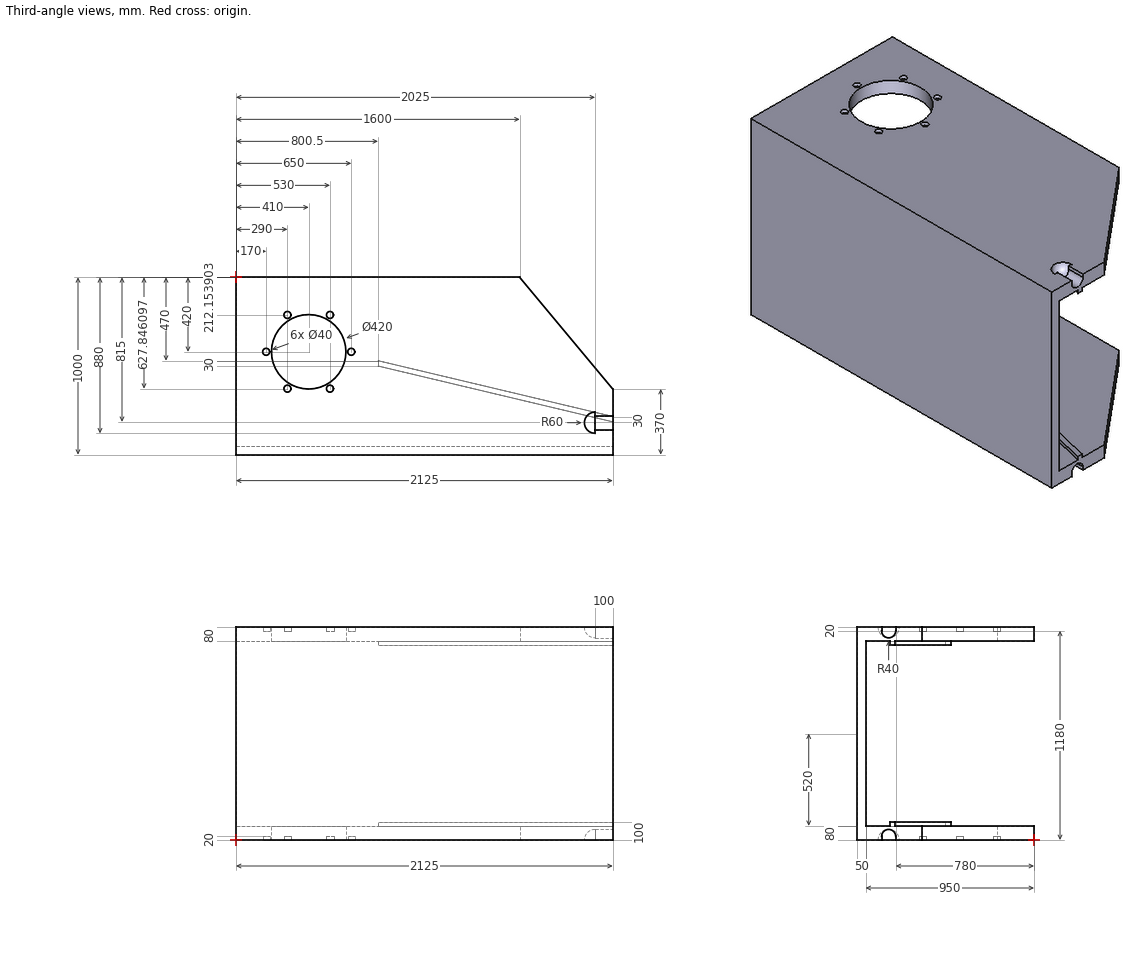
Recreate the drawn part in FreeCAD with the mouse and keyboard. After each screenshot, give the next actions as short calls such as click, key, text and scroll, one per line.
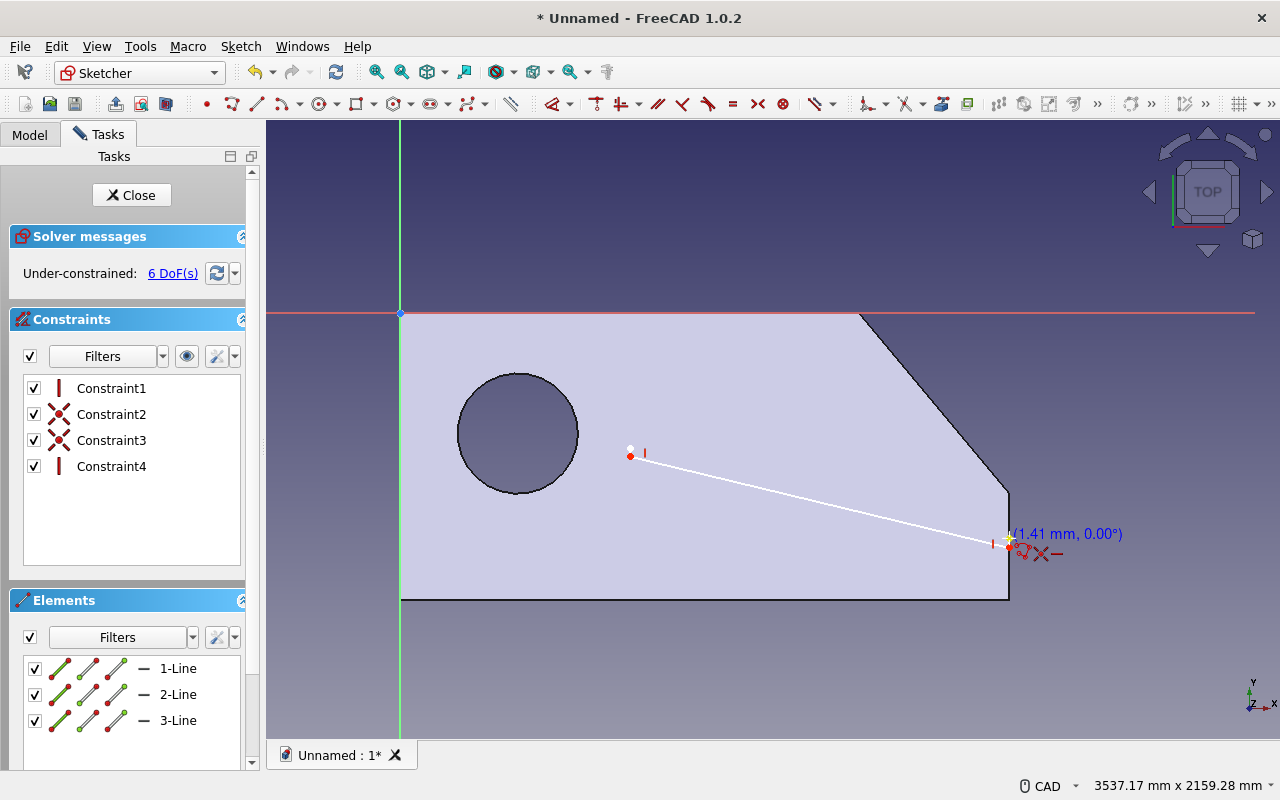
scroll(630, 448, up, 7)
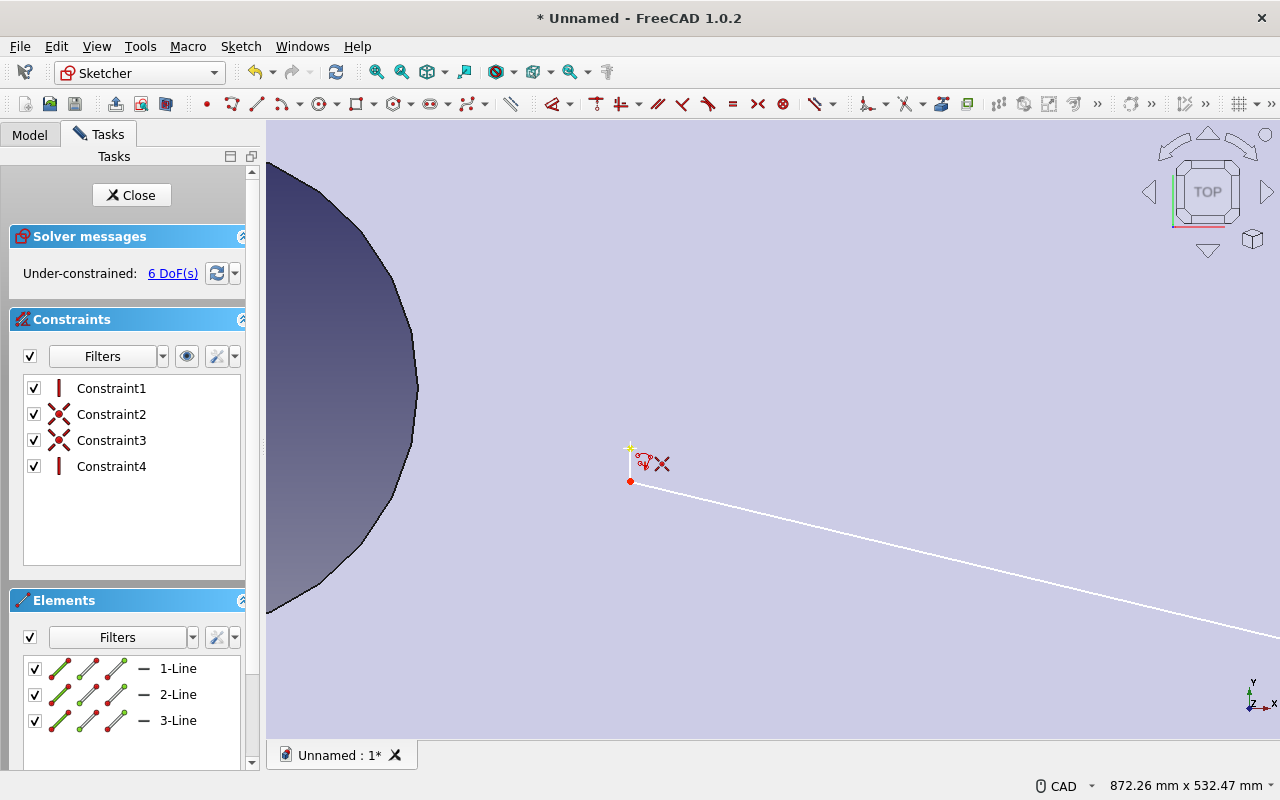
click(630, 449)
key(Escape)
key(Escape)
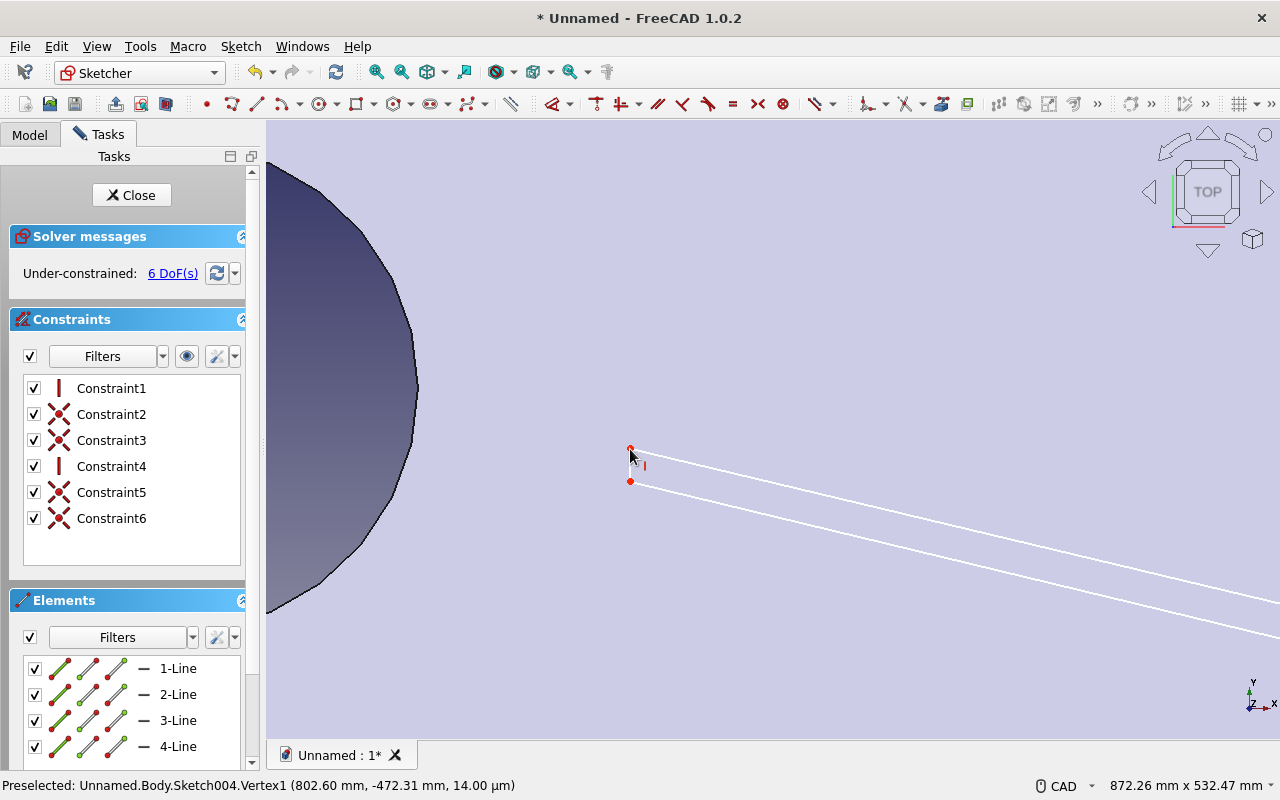
key(d)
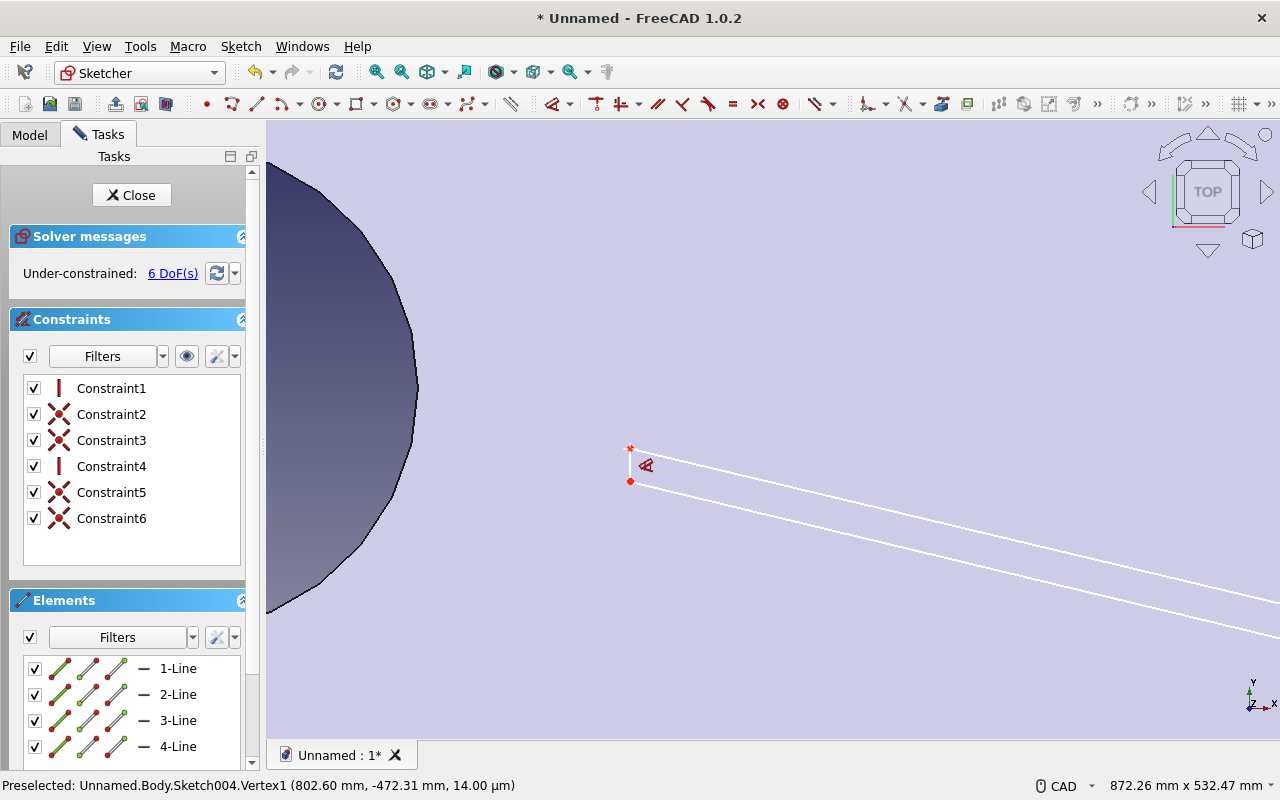
scroll(630, 459, up, 2)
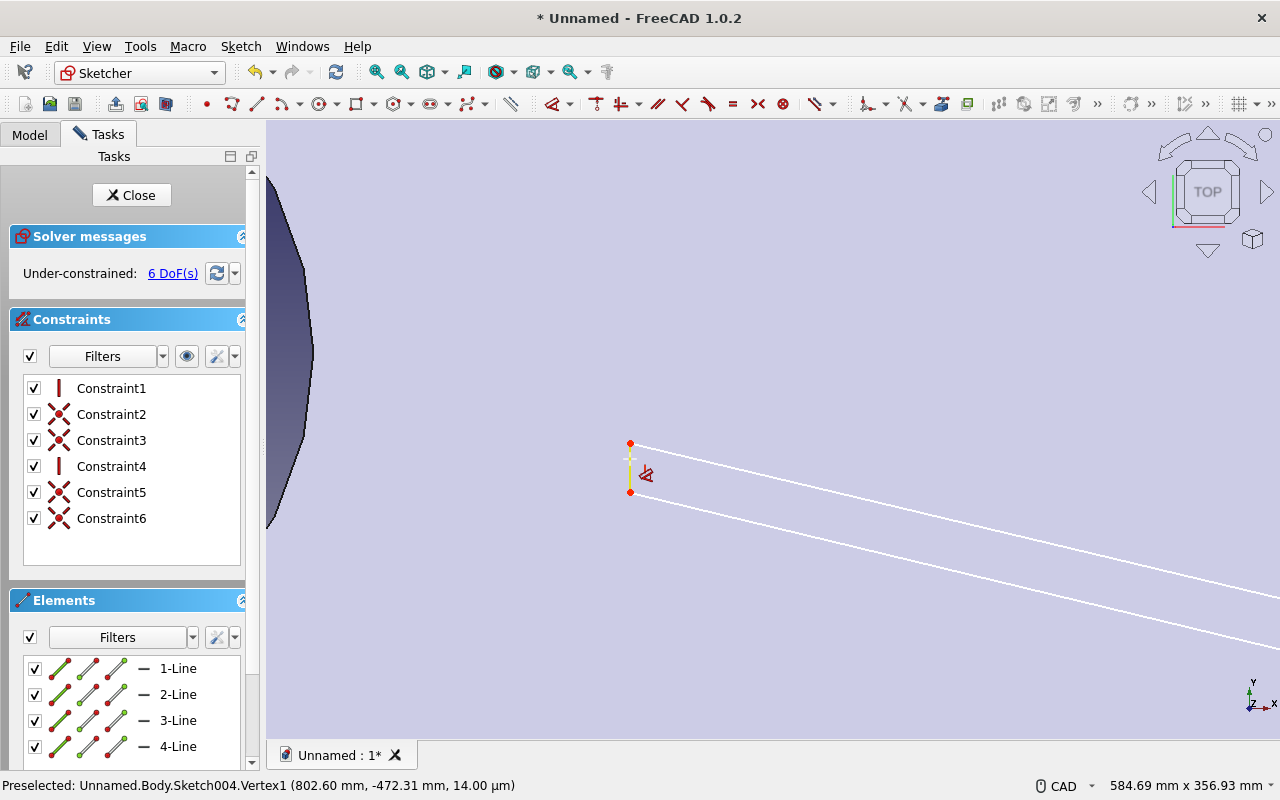
click(630, 458)
click(596, 468)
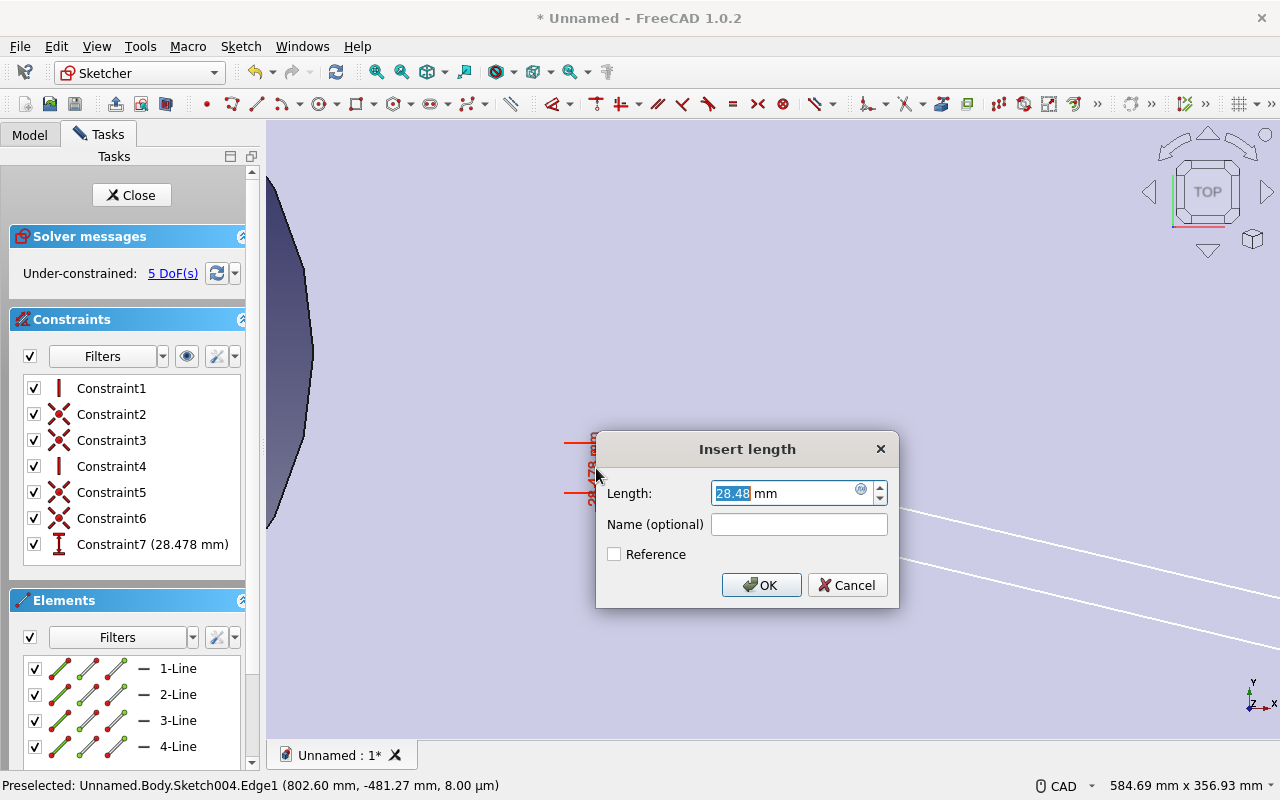
text(30)
key(Return)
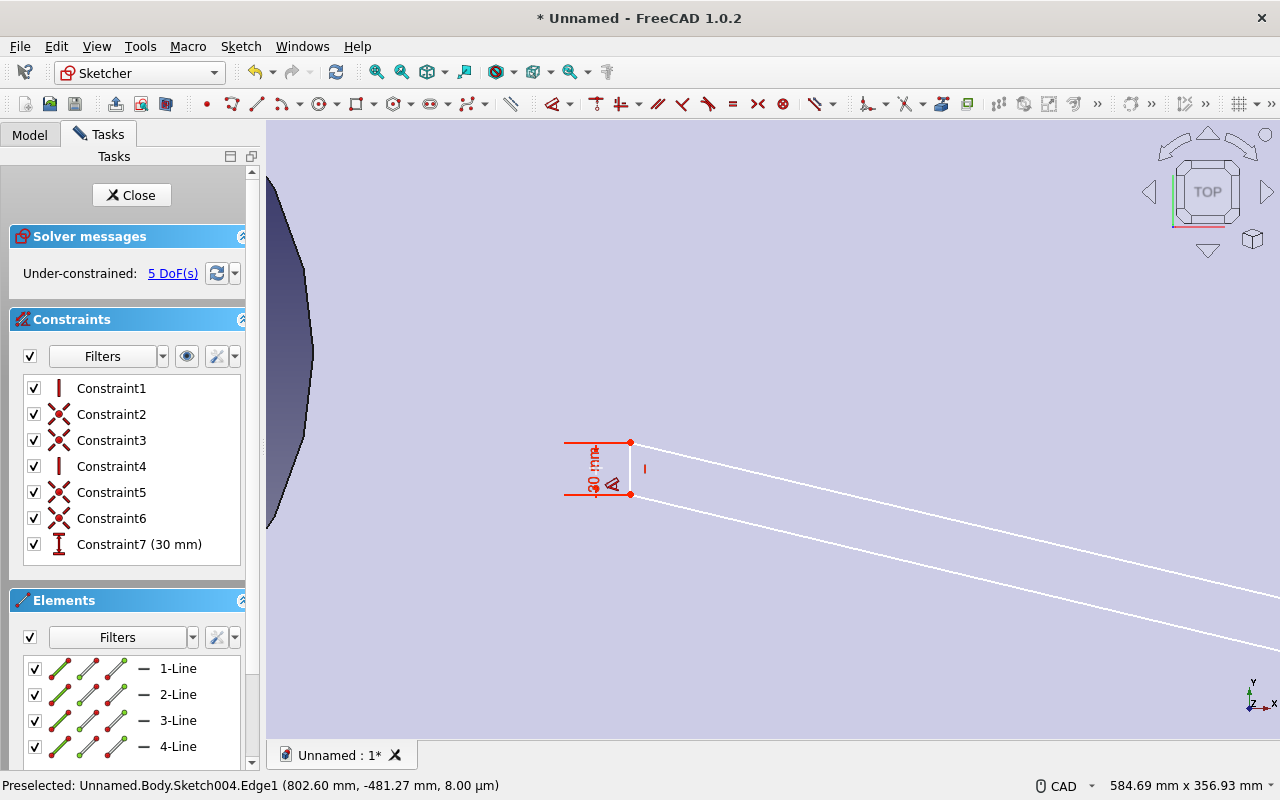
scroll(630, 449, down, 9)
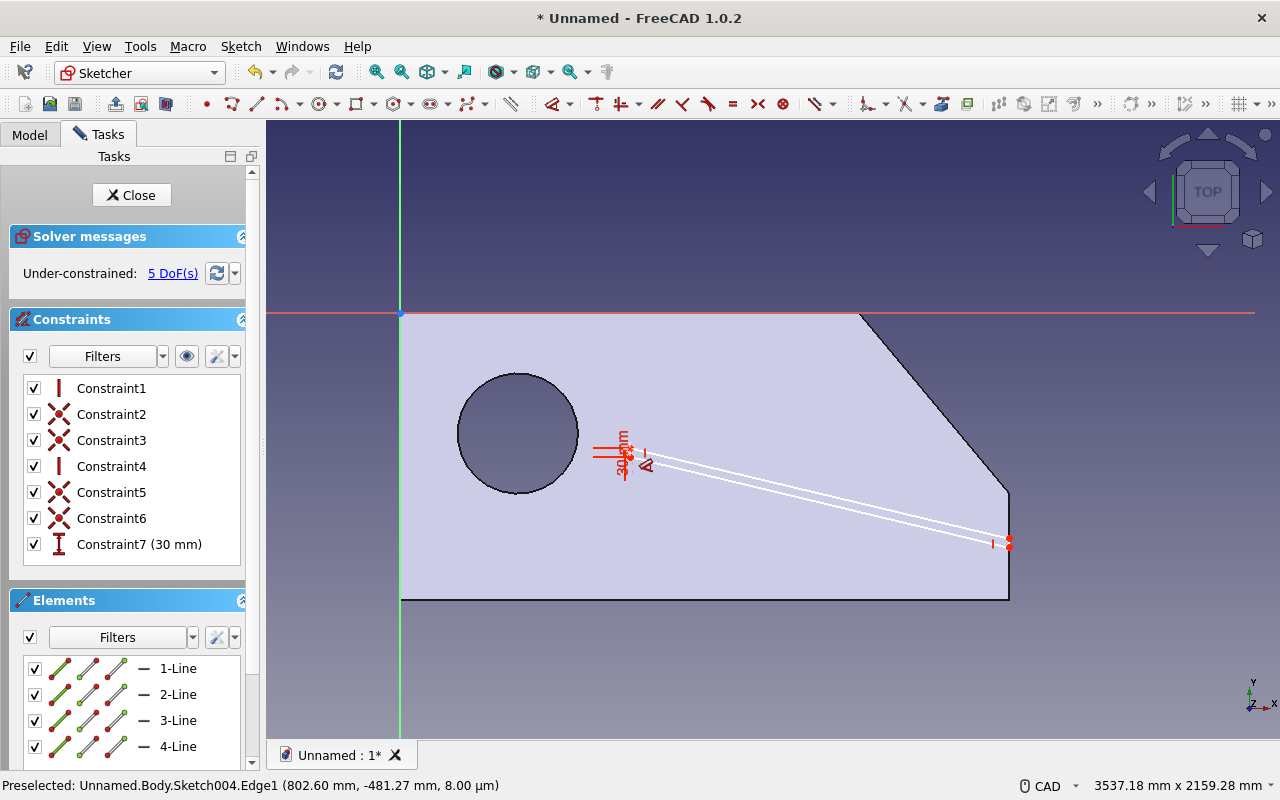
scroll(1009, 545, up, 9)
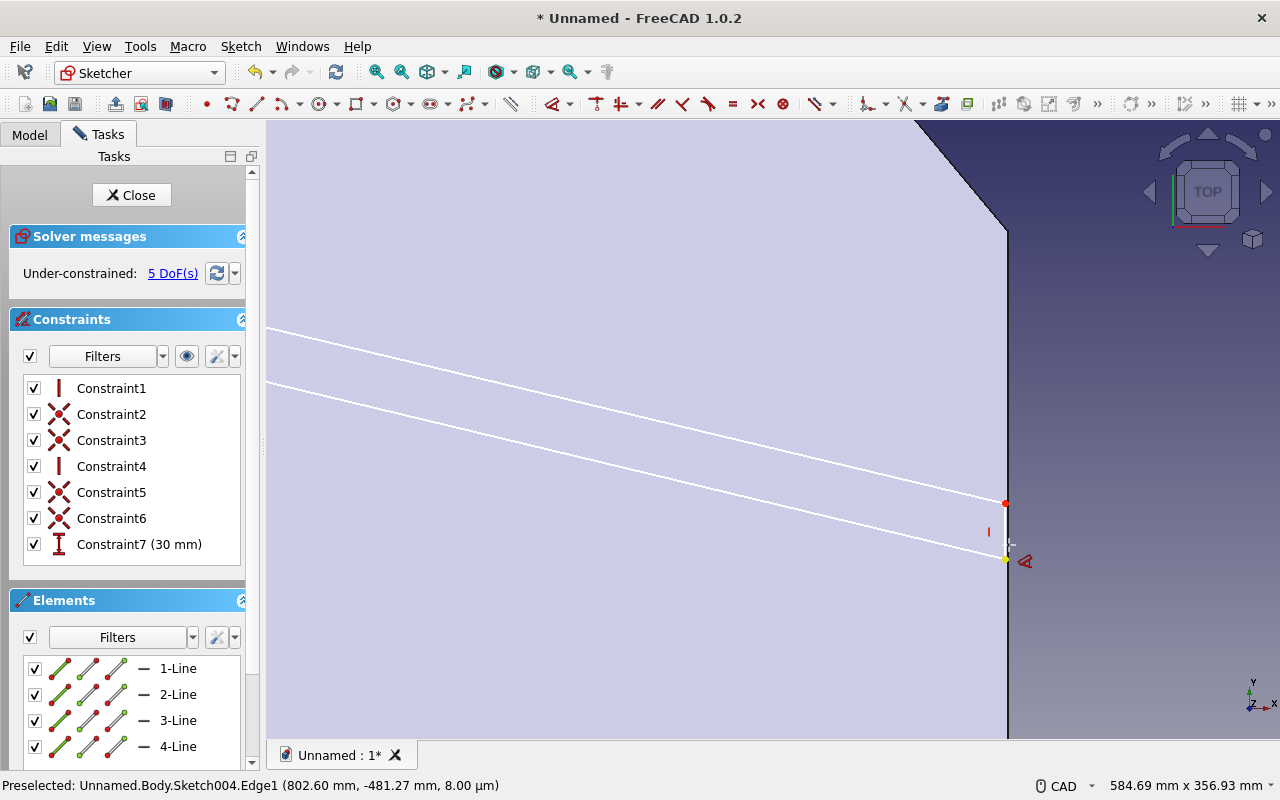
click(1005, 543)
click(1039, 532)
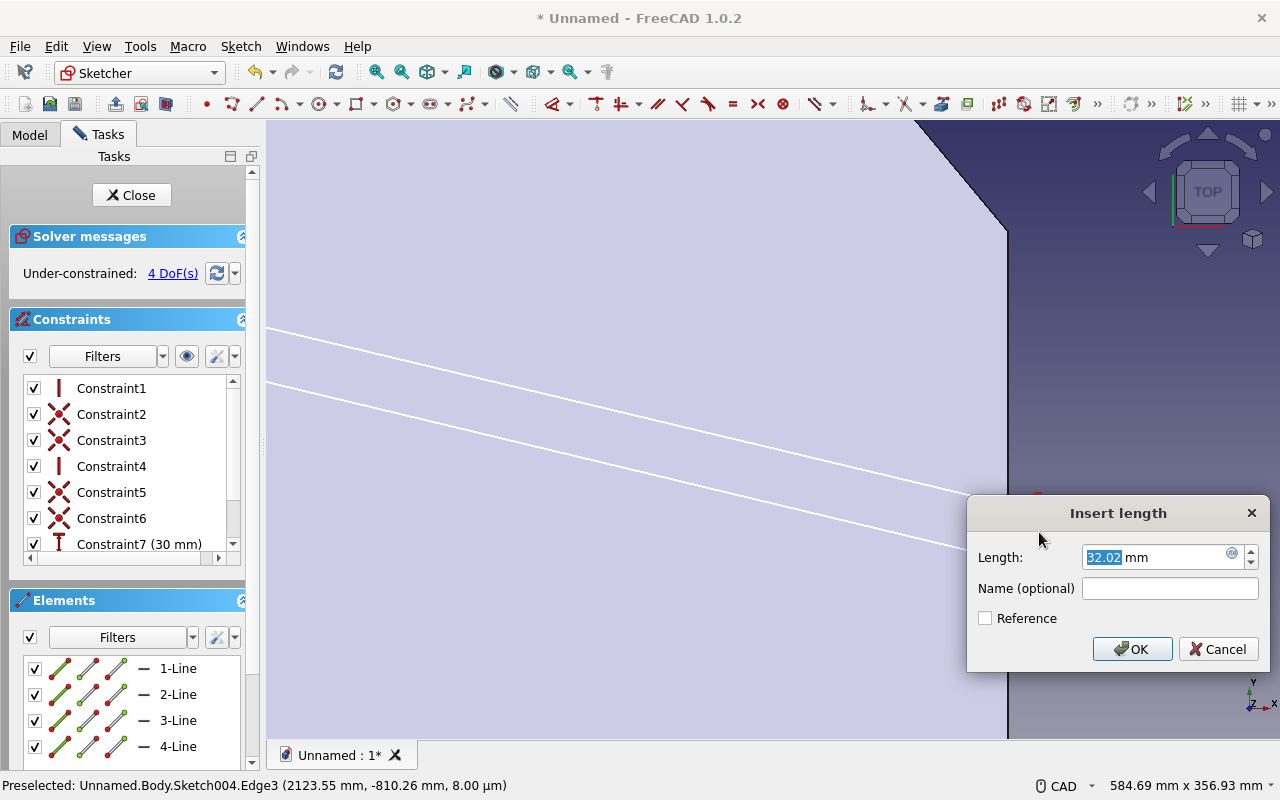
text(30)
key(Return)